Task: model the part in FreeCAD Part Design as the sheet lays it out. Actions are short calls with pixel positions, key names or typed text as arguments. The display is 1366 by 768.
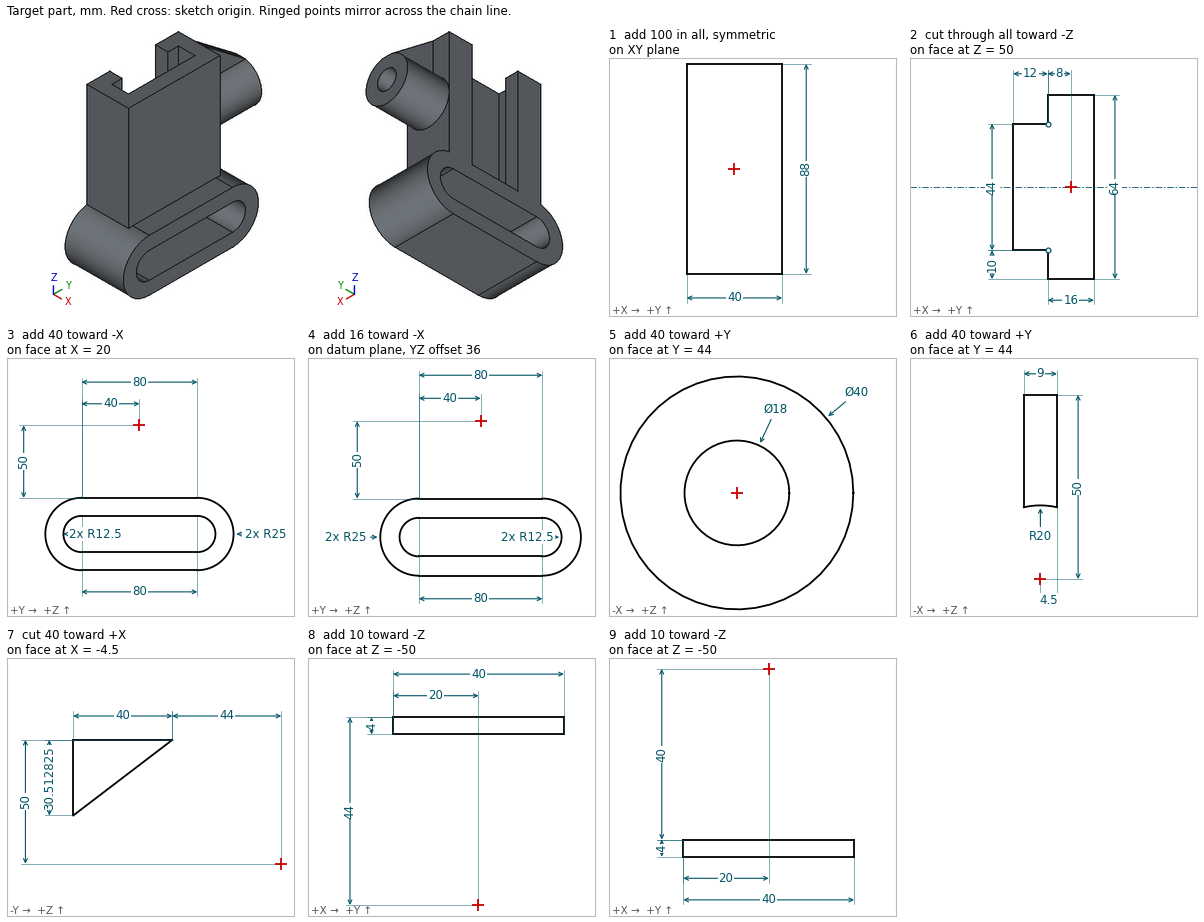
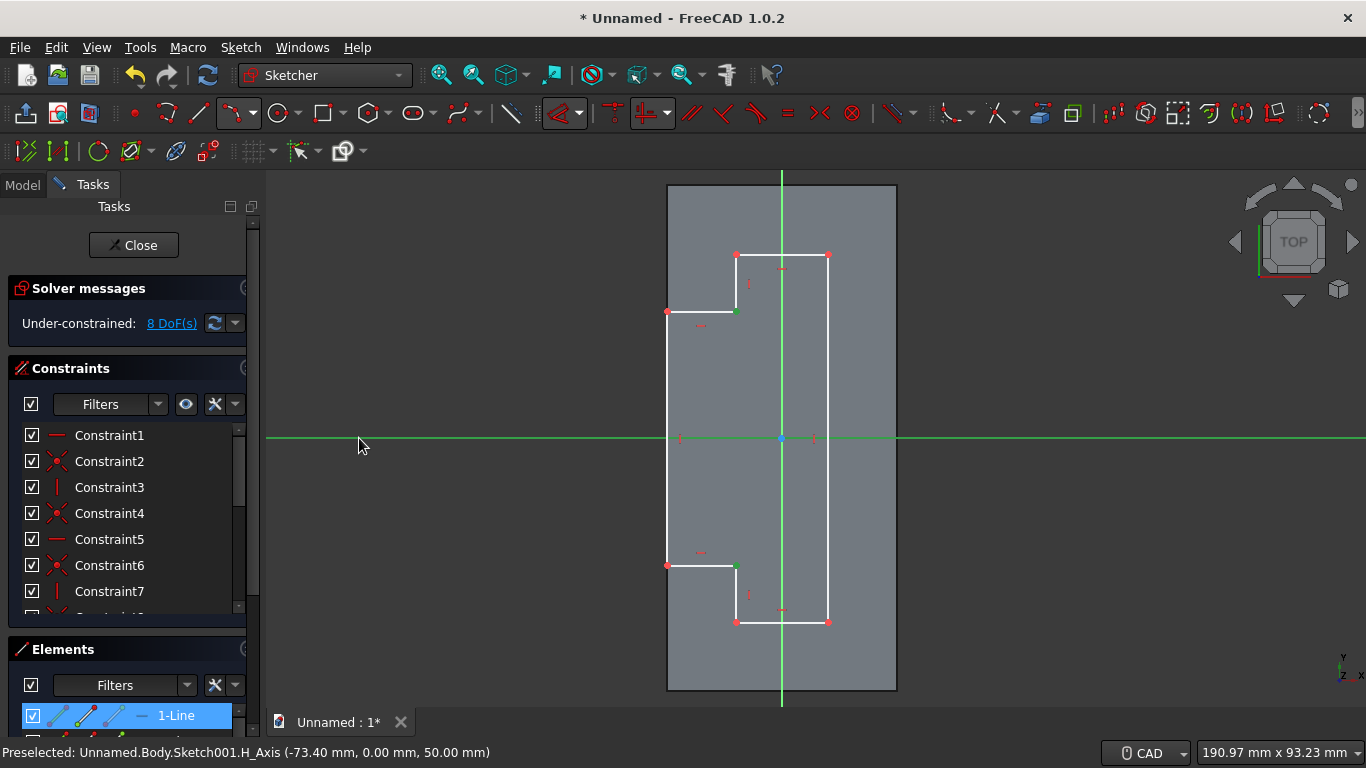
key(s)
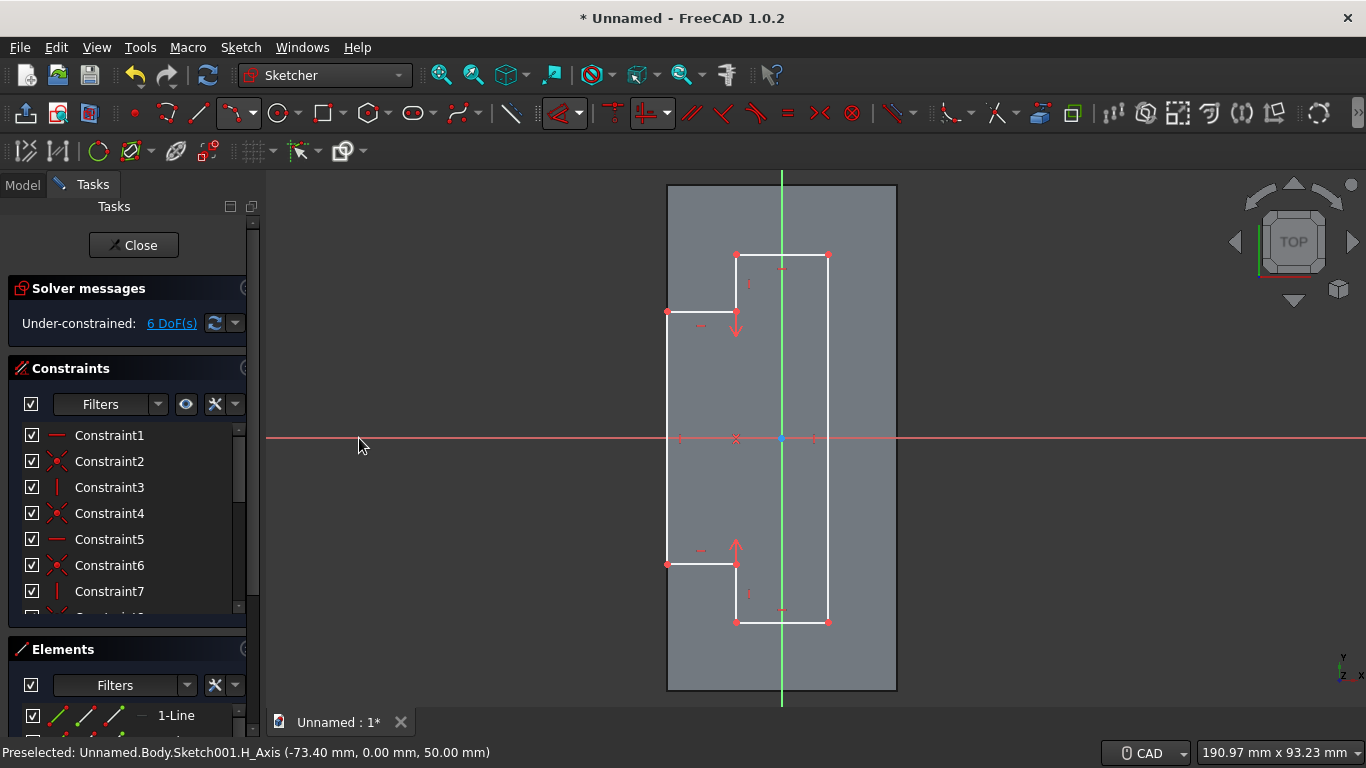
click(715, 312)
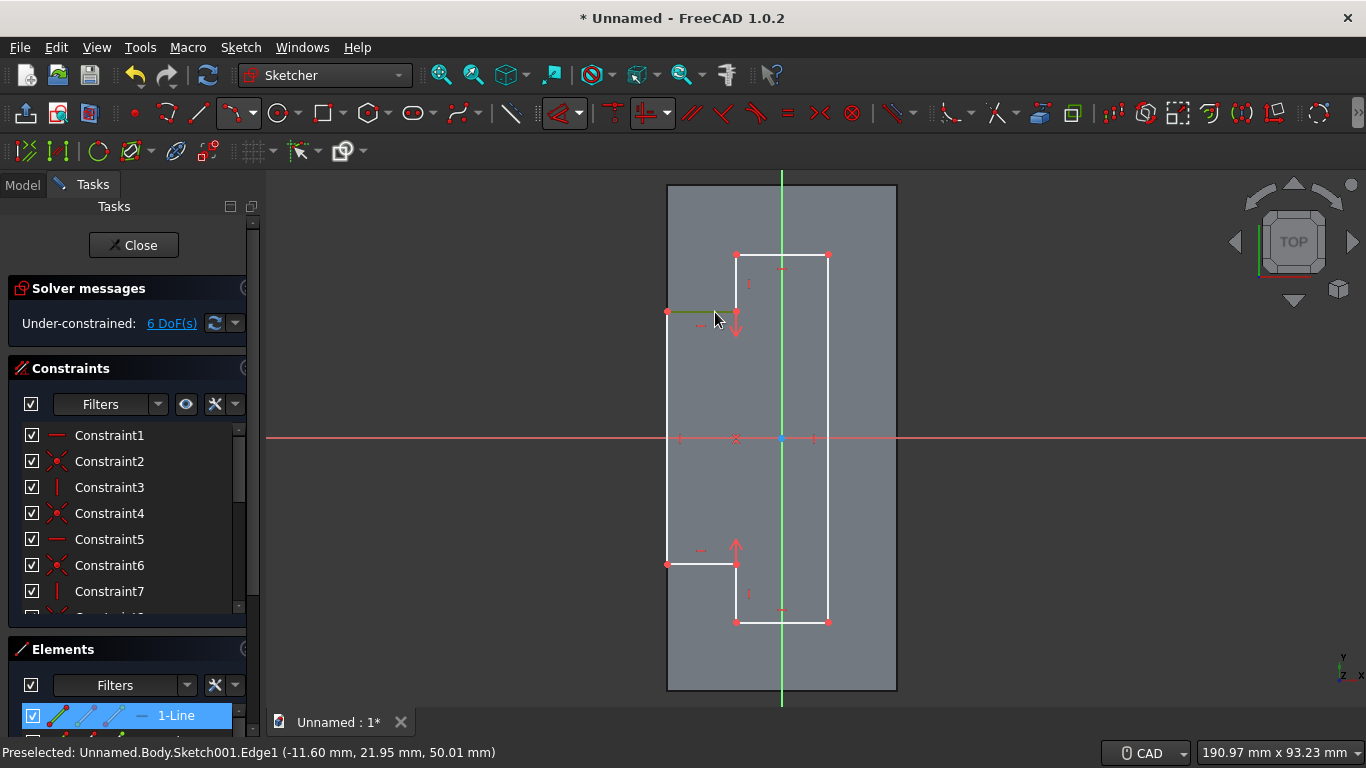
click(582, 114)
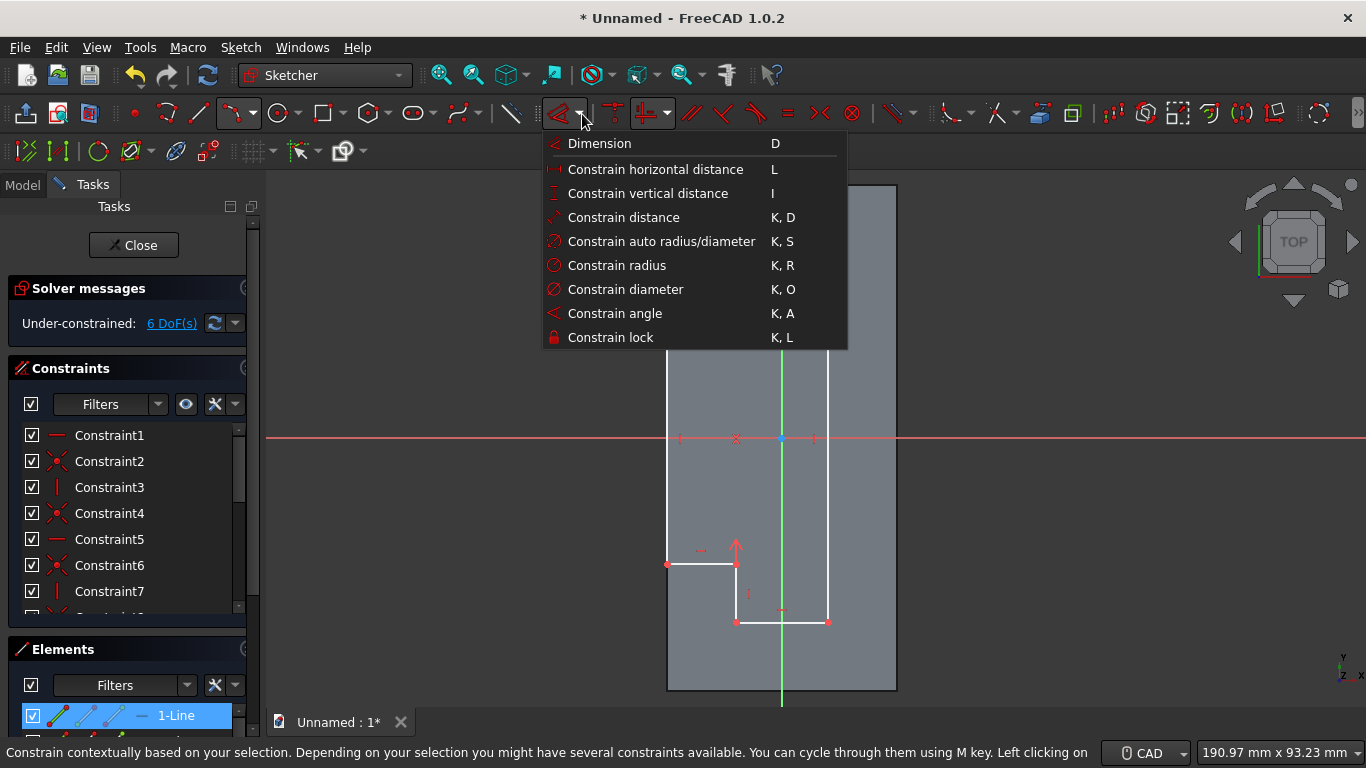
click(695, 169)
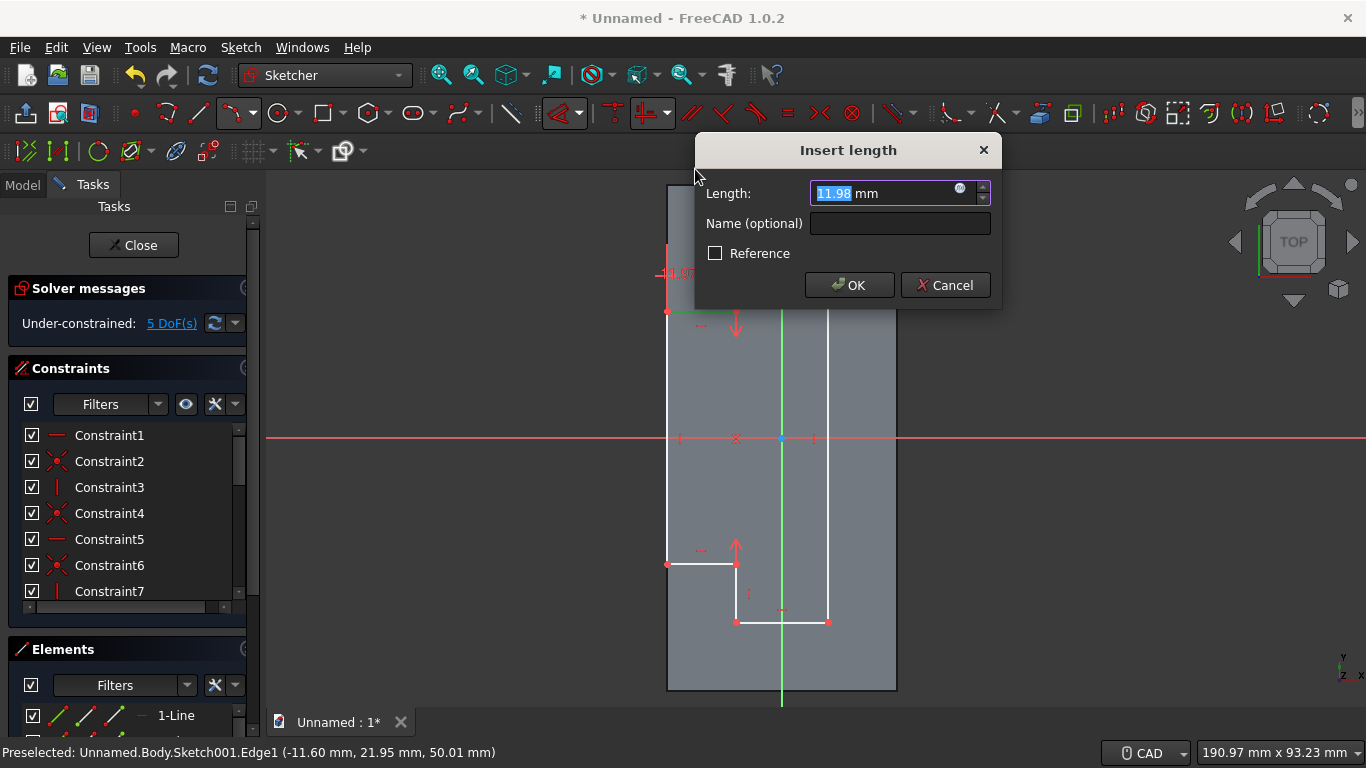
text(12)
key(Return)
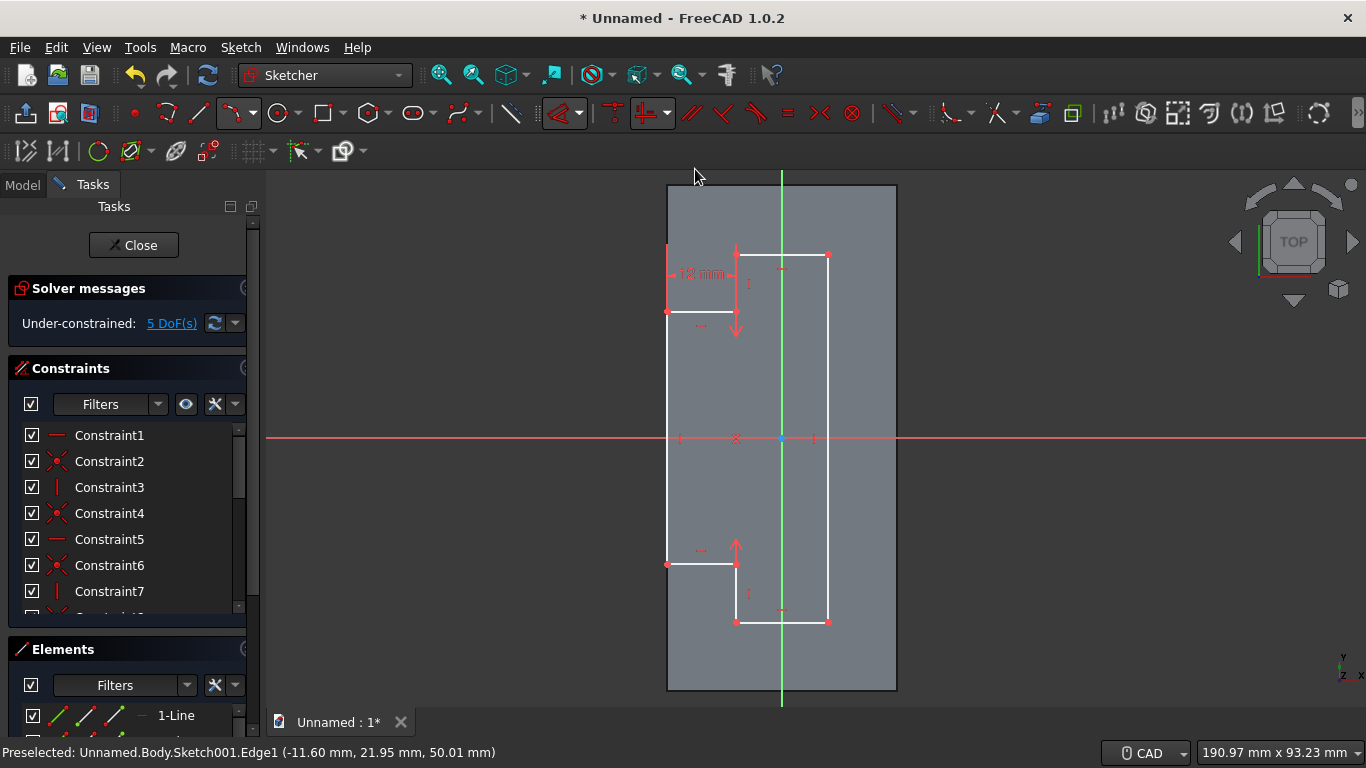
click(667, 387)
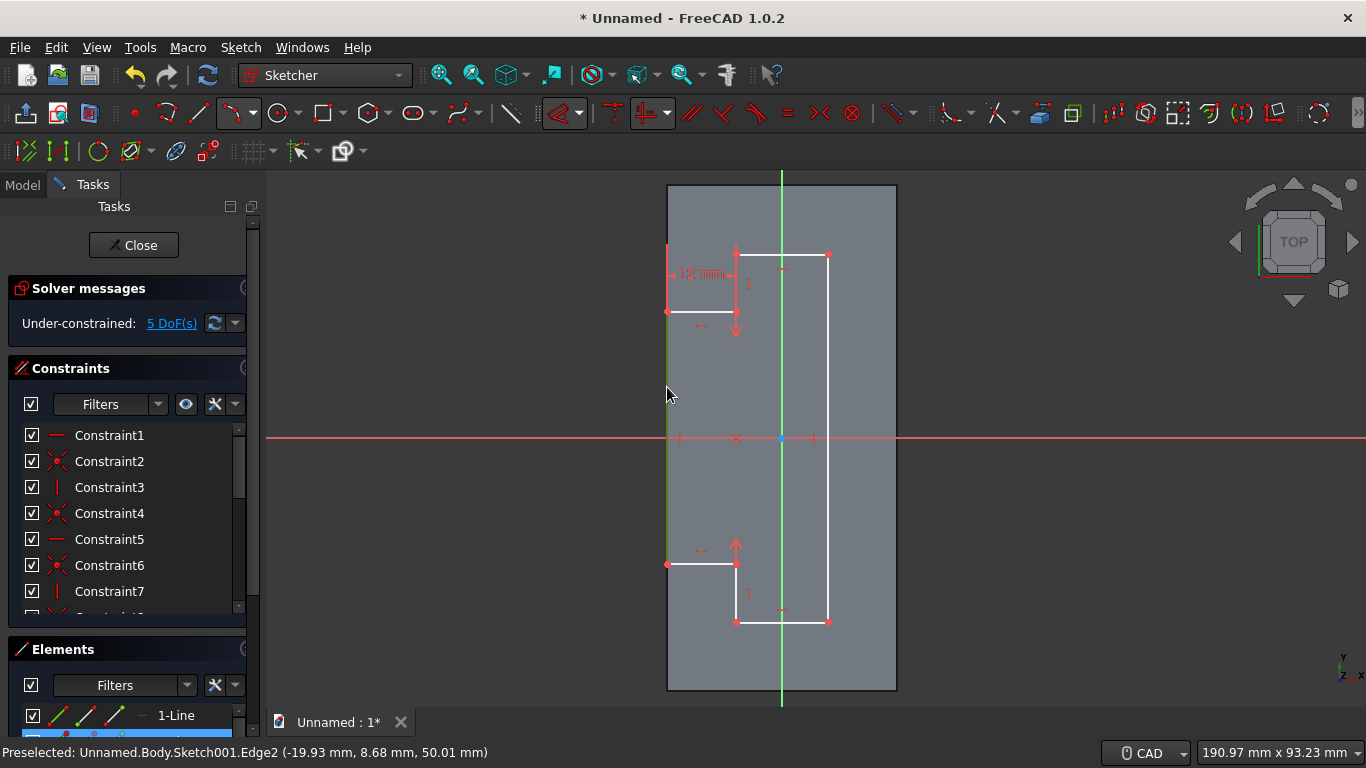
key(i)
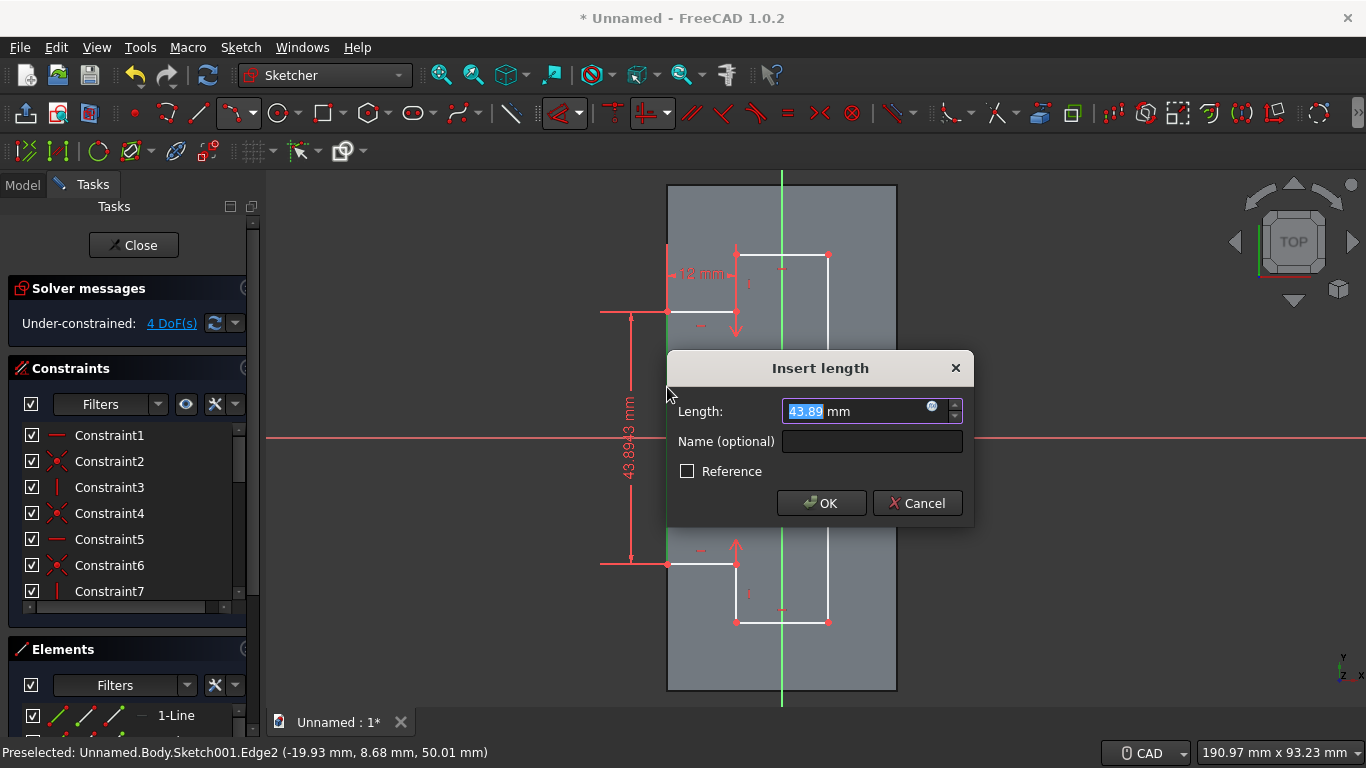
text(44)
key(Return)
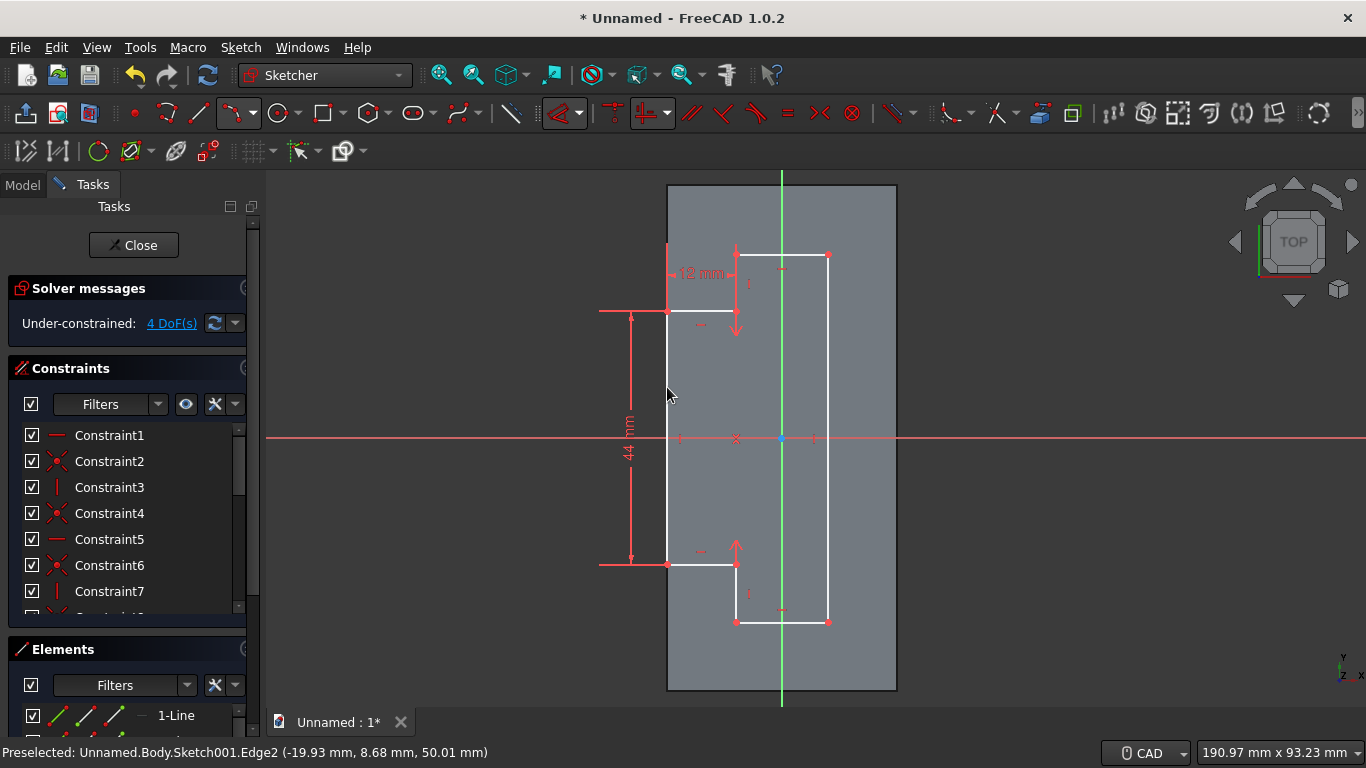
click(736, 582)